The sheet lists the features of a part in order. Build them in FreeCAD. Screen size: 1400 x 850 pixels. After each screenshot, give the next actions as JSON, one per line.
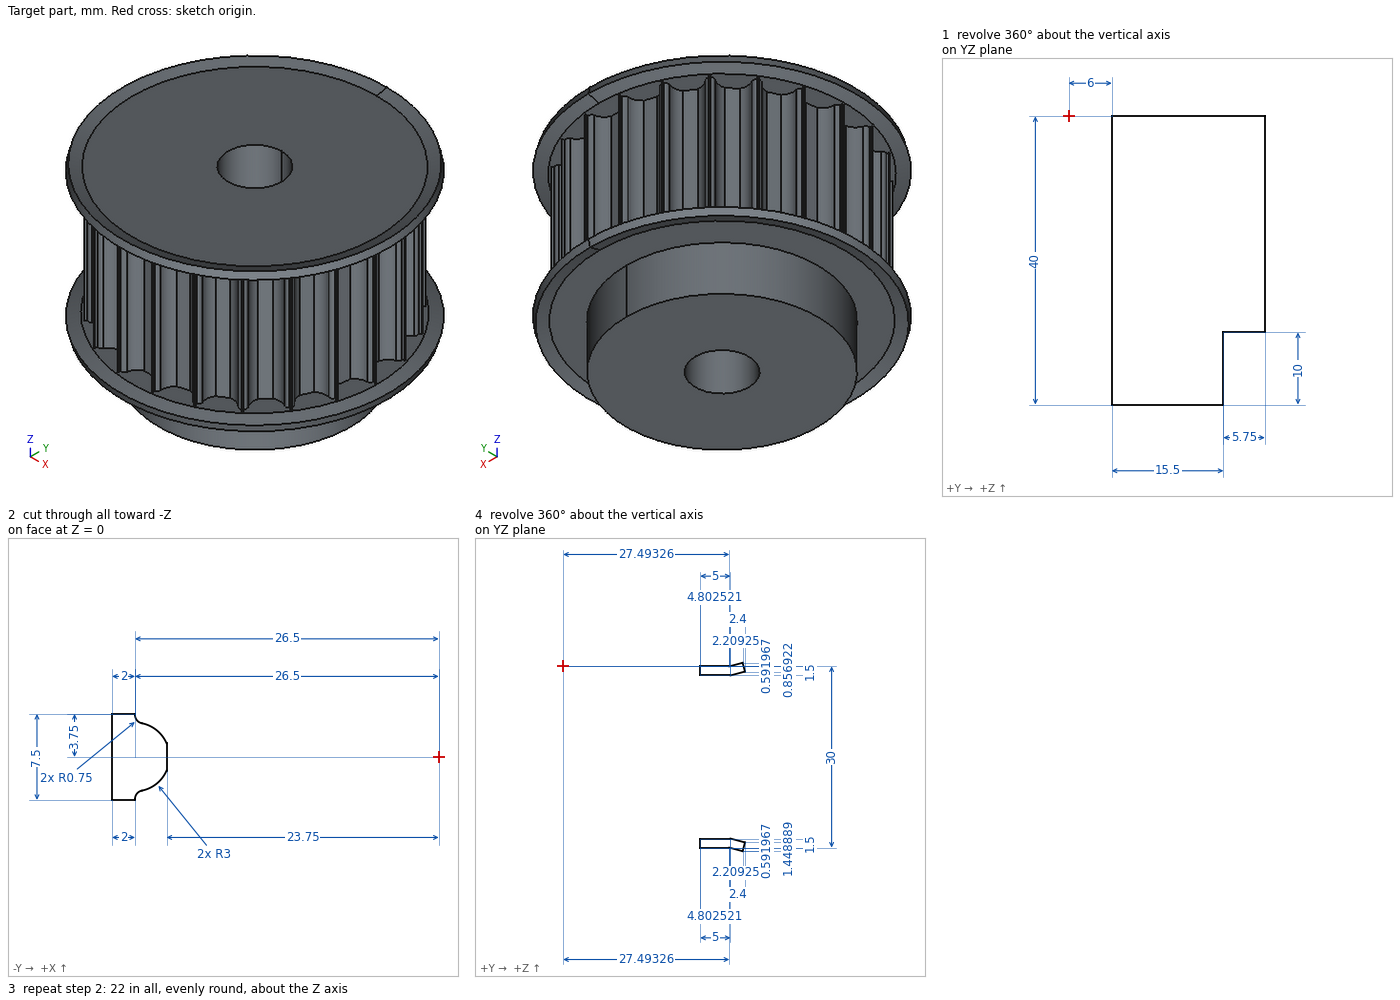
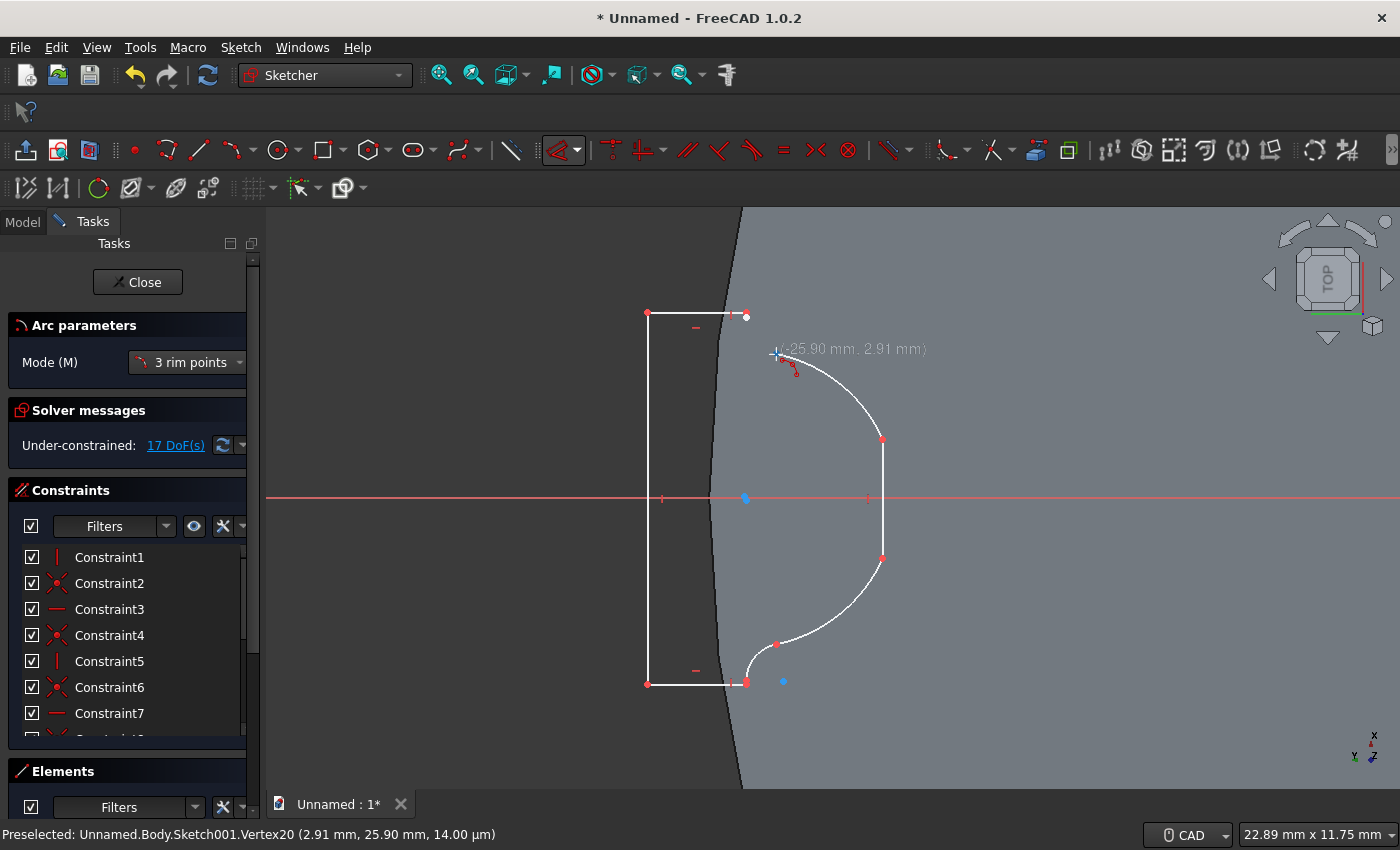
{"action": "scroll", "coordinate": [746, 316], "scroll_direction": "up", "scroll_amount": 11}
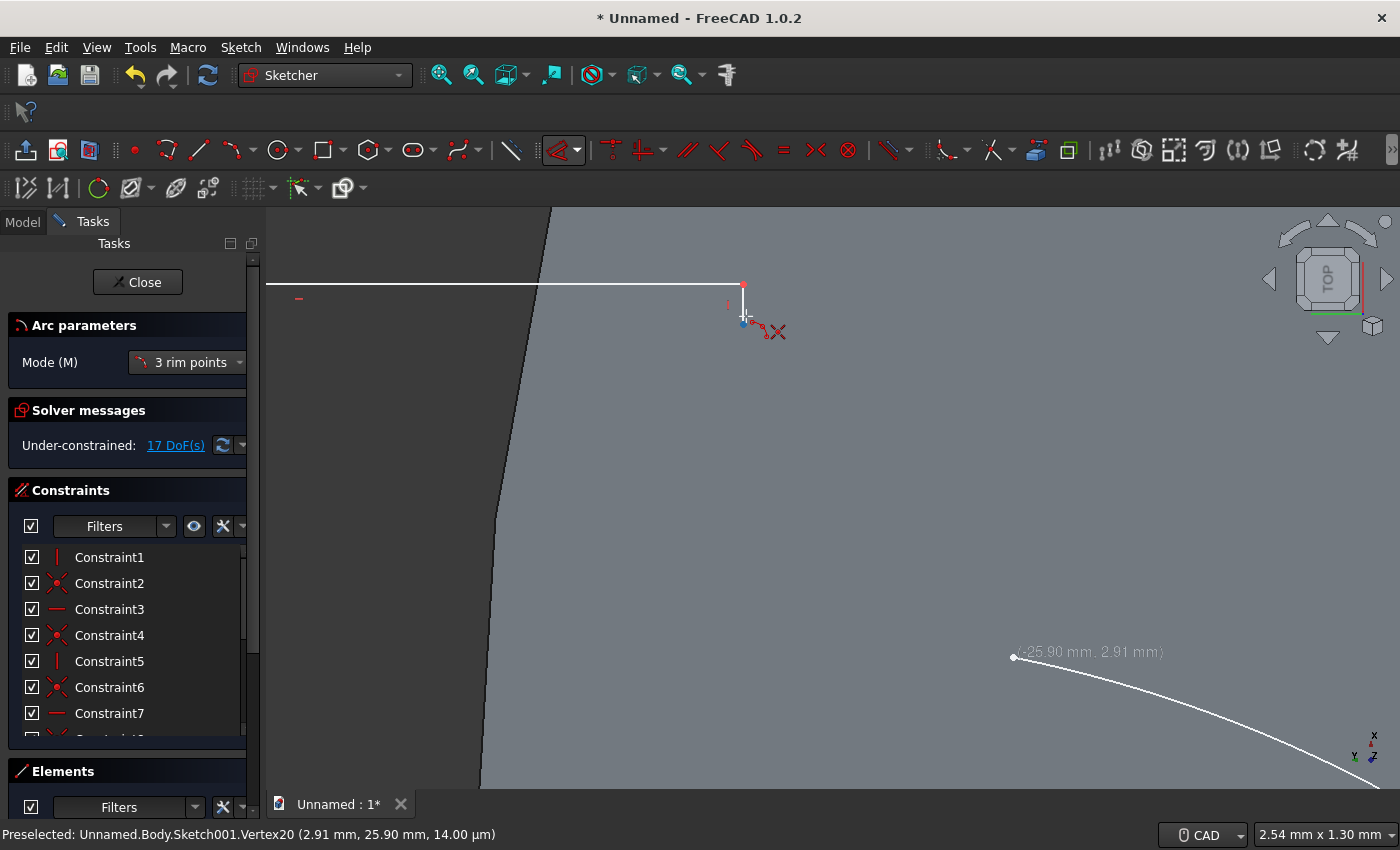
{"action": "left_click", "coordinate": [743, 324]}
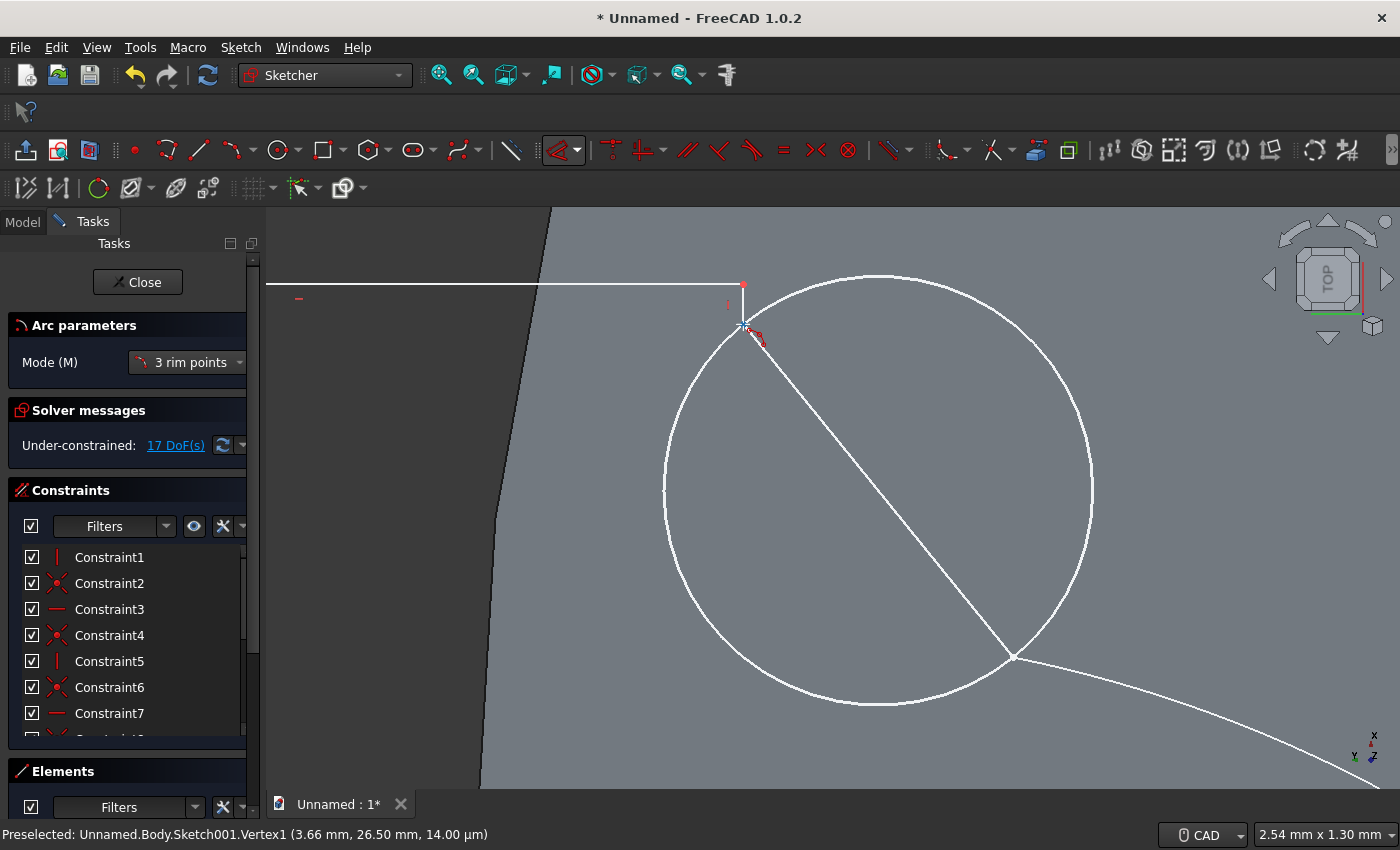
{"action": "scroll", "coordinate": [746, 316], "scroll_direction": "down", "scroll_amount": 11}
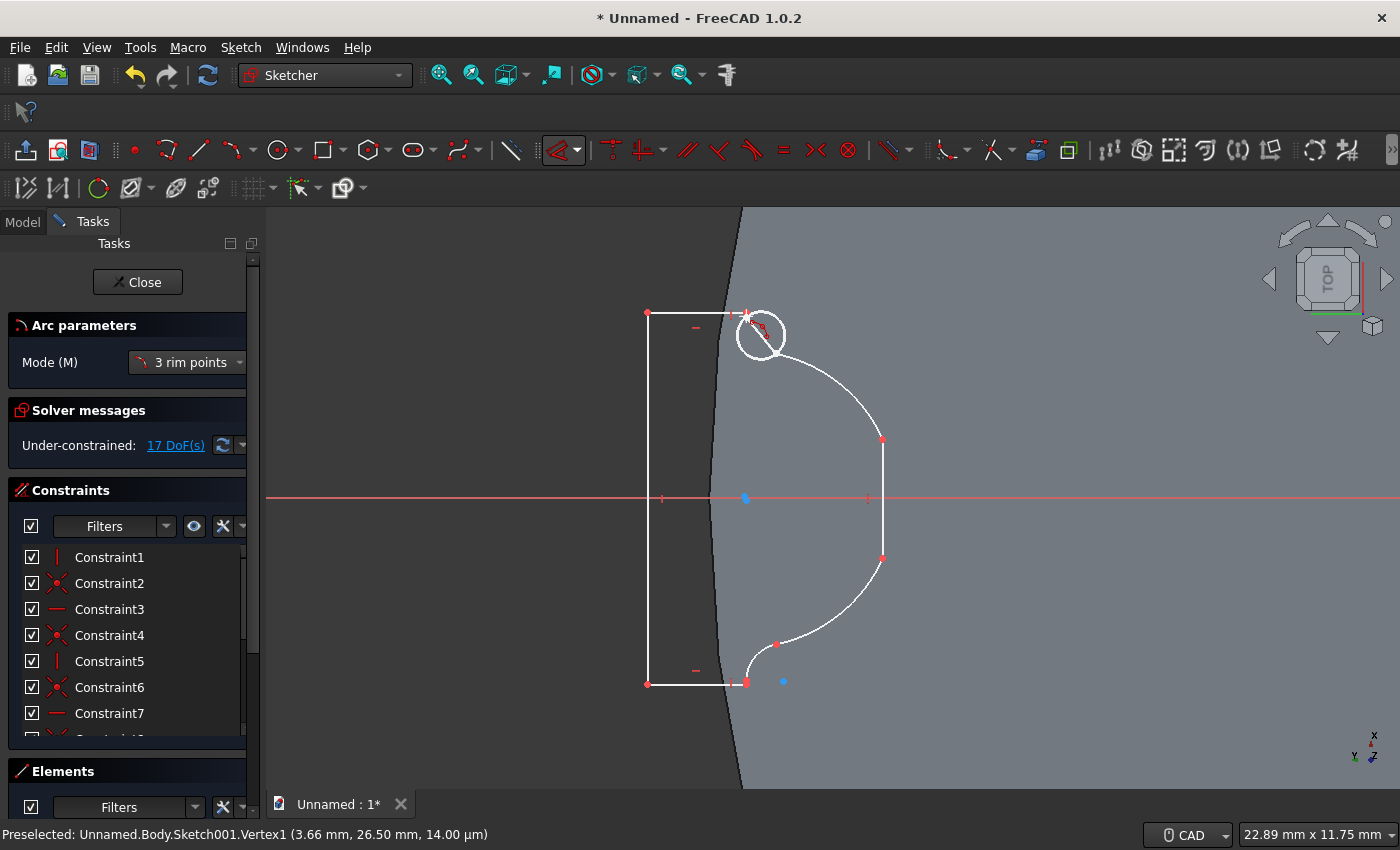
{"action": "scroll", "coordinate": [755, 340], "scroll_direction": "up", "scroll_amount": 4}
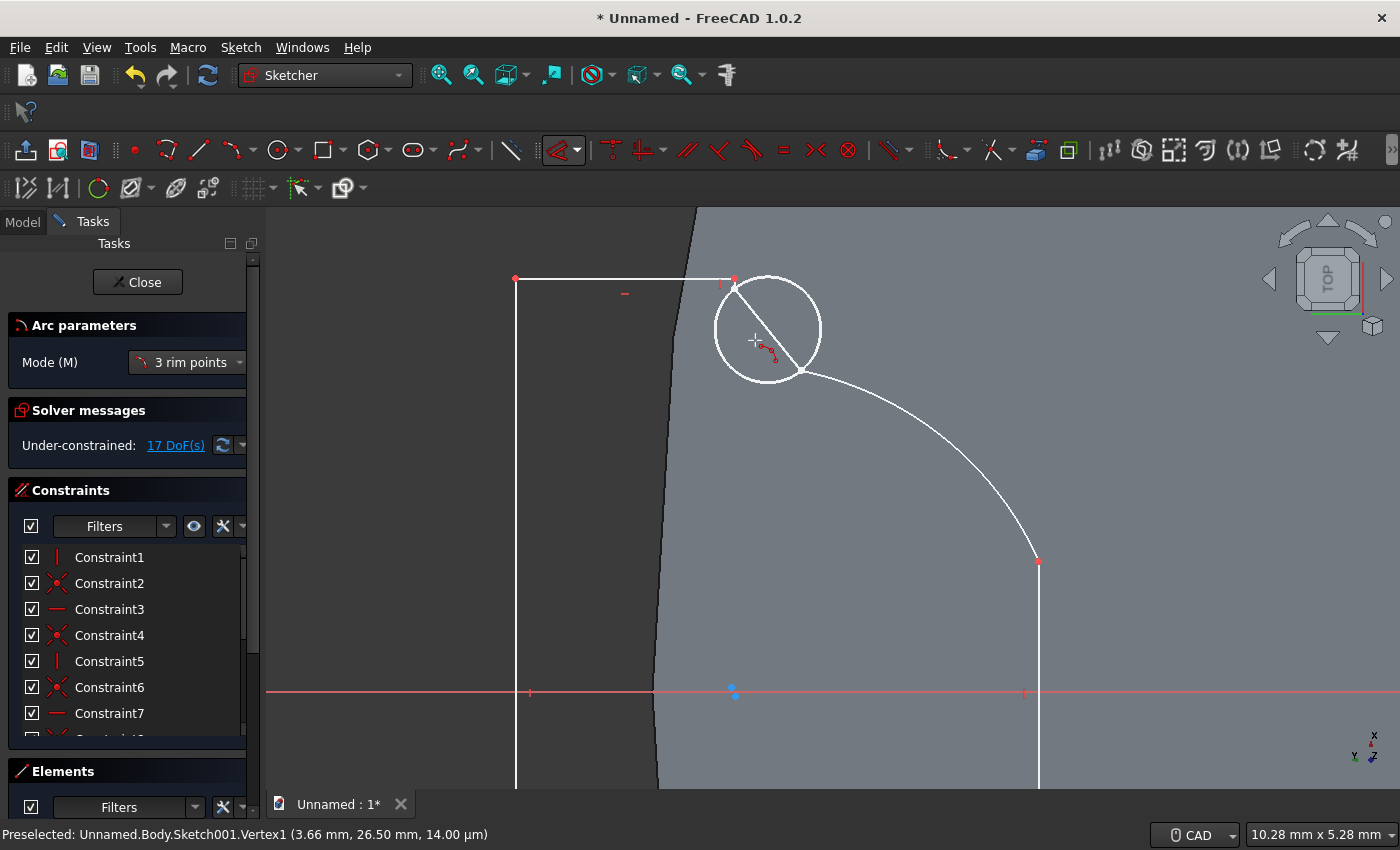
{"action": "left_click", "coordinate": [754, 339]}
{"action": "key", "text": "Escape"}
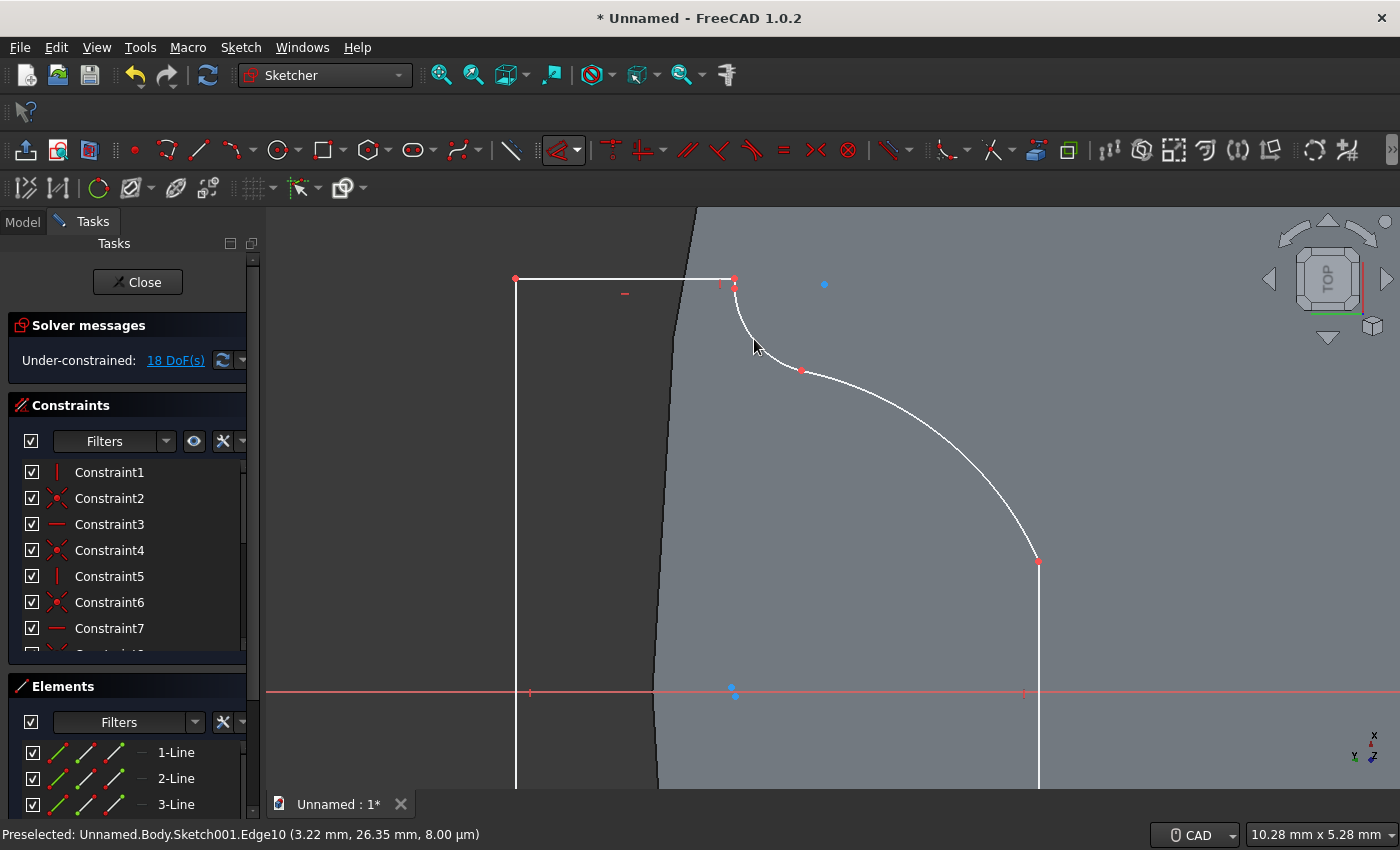
{"action": "scroll", "coordinate": [735, 284], "scroll_direction": "up", "scroll_amount": 6}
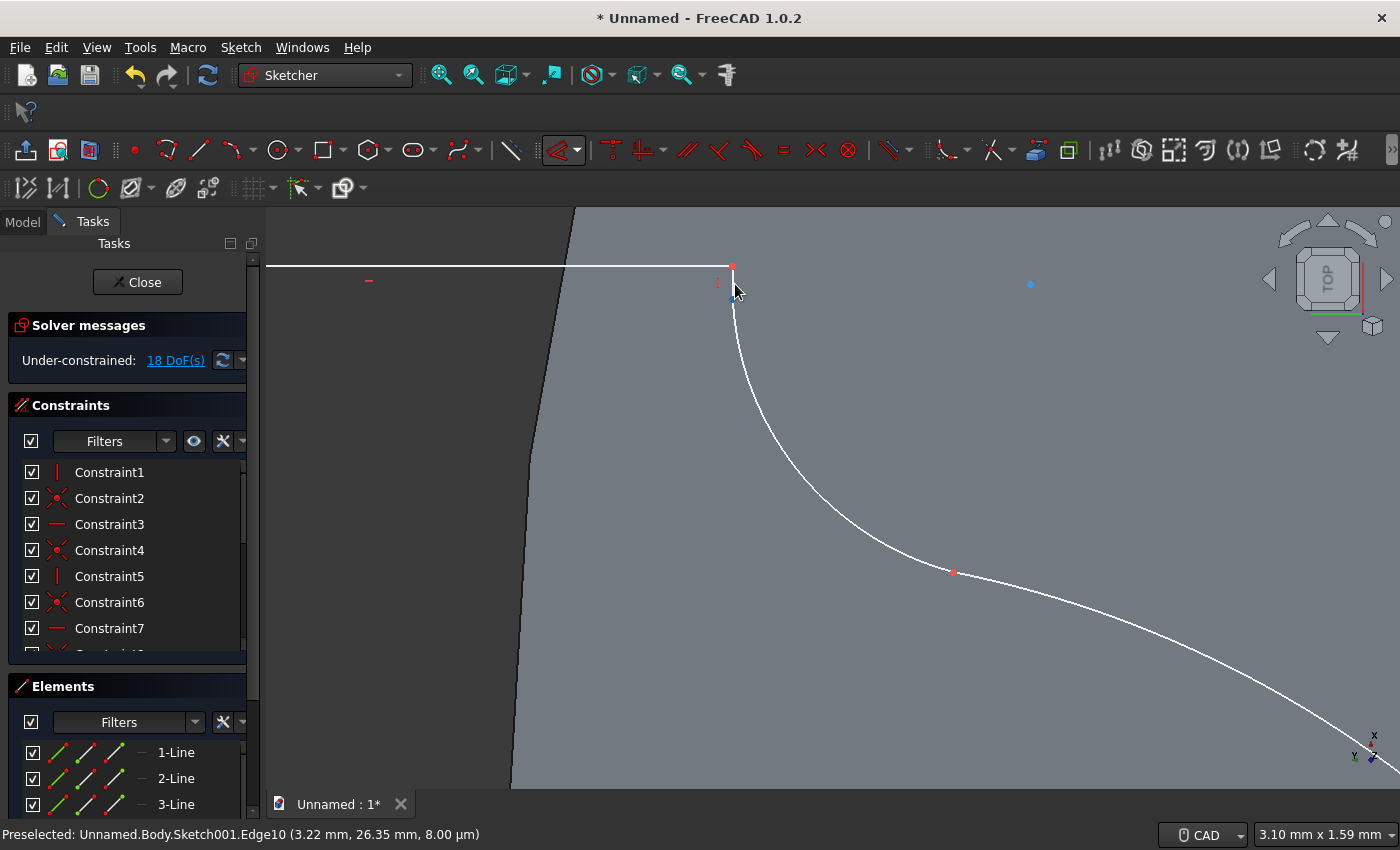
{"action": "left_click", "coordinate": [733, 283]}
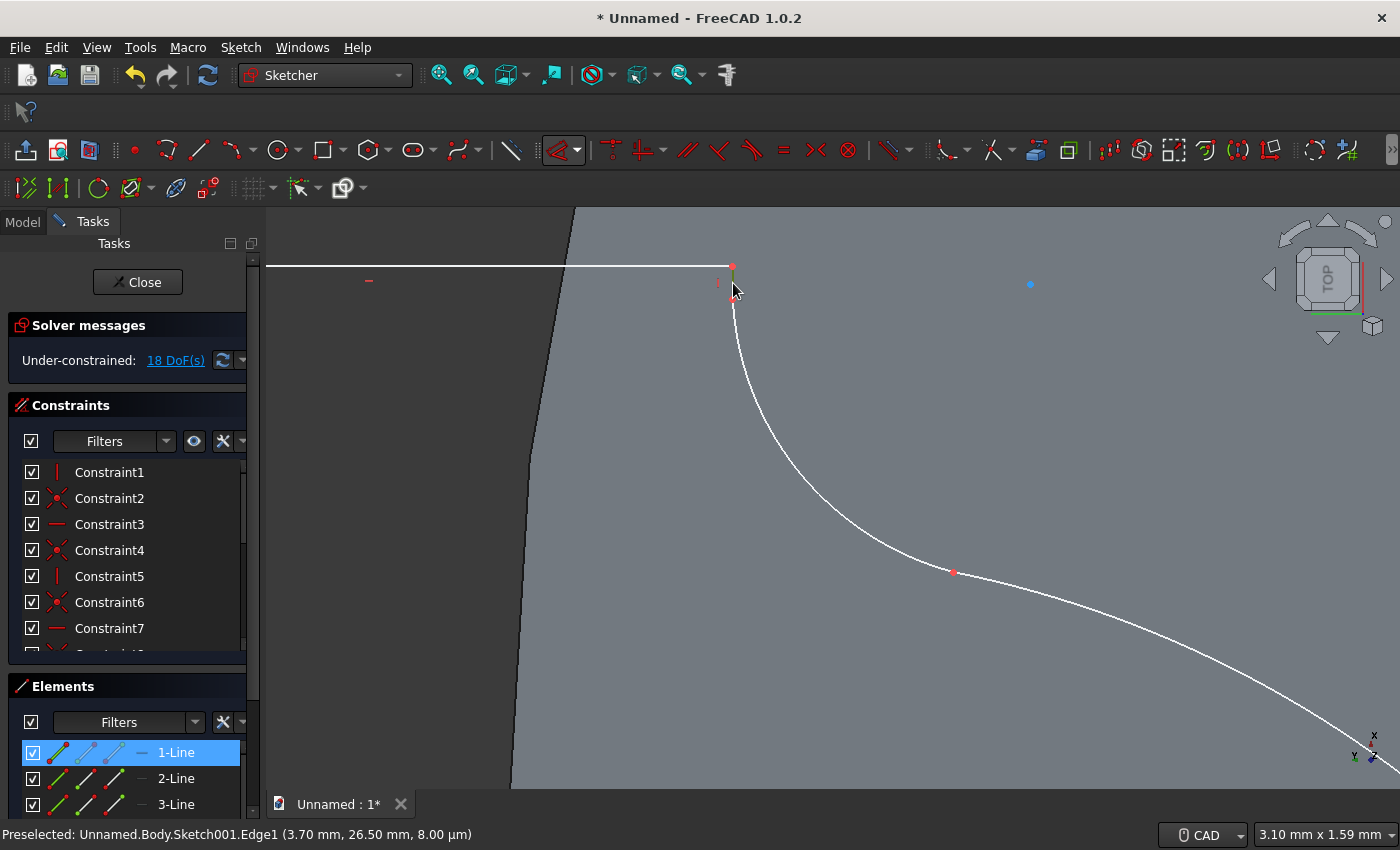
{"action": "scroll", "coordinate": [748, 320], "scroll_direction": "down", "scroll_amount": 10}